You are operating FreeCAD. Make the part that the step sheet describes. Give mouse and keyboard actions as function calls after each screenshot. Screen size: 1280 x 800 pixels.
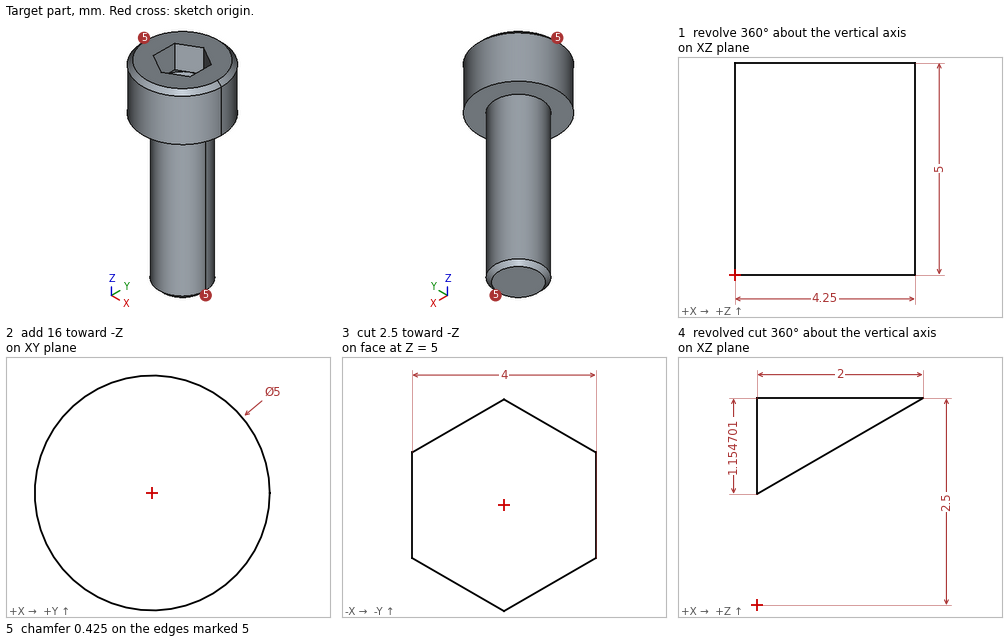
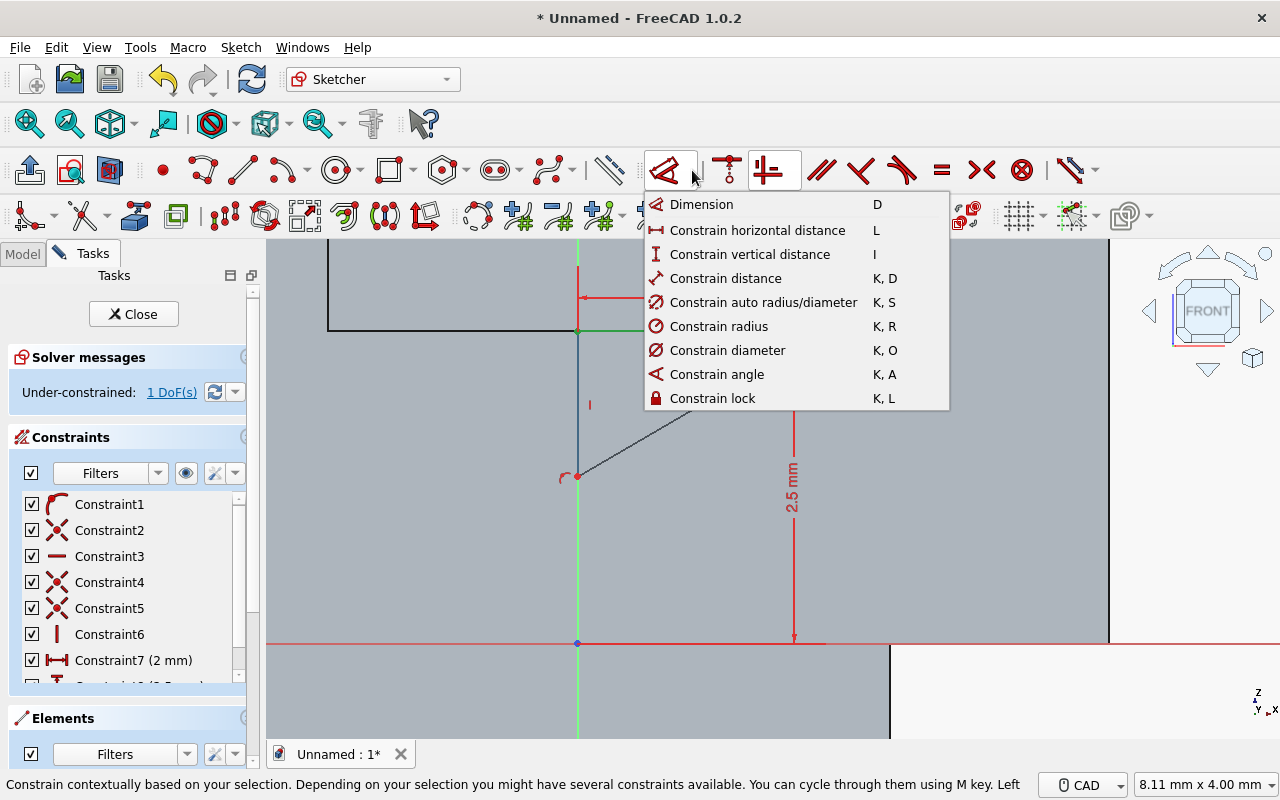
click(797, 254)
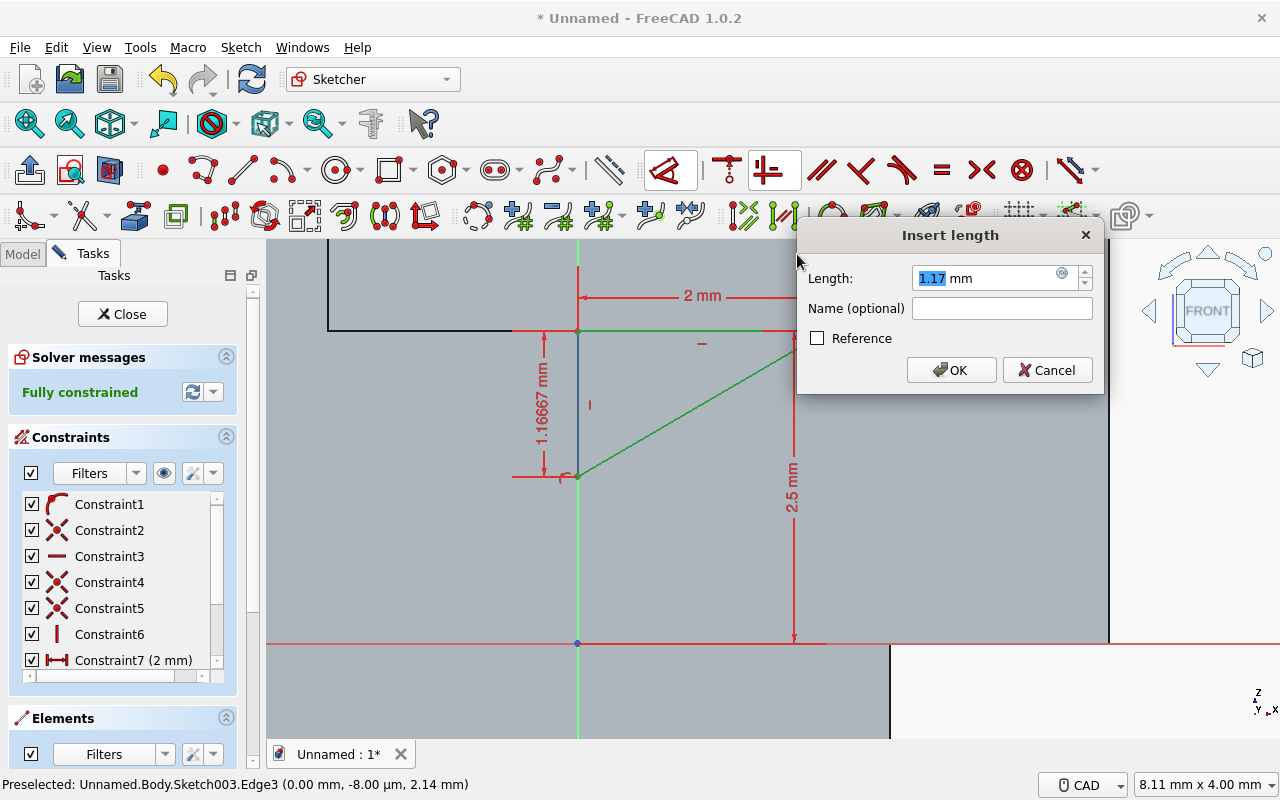
text(1.154701)
key(Return)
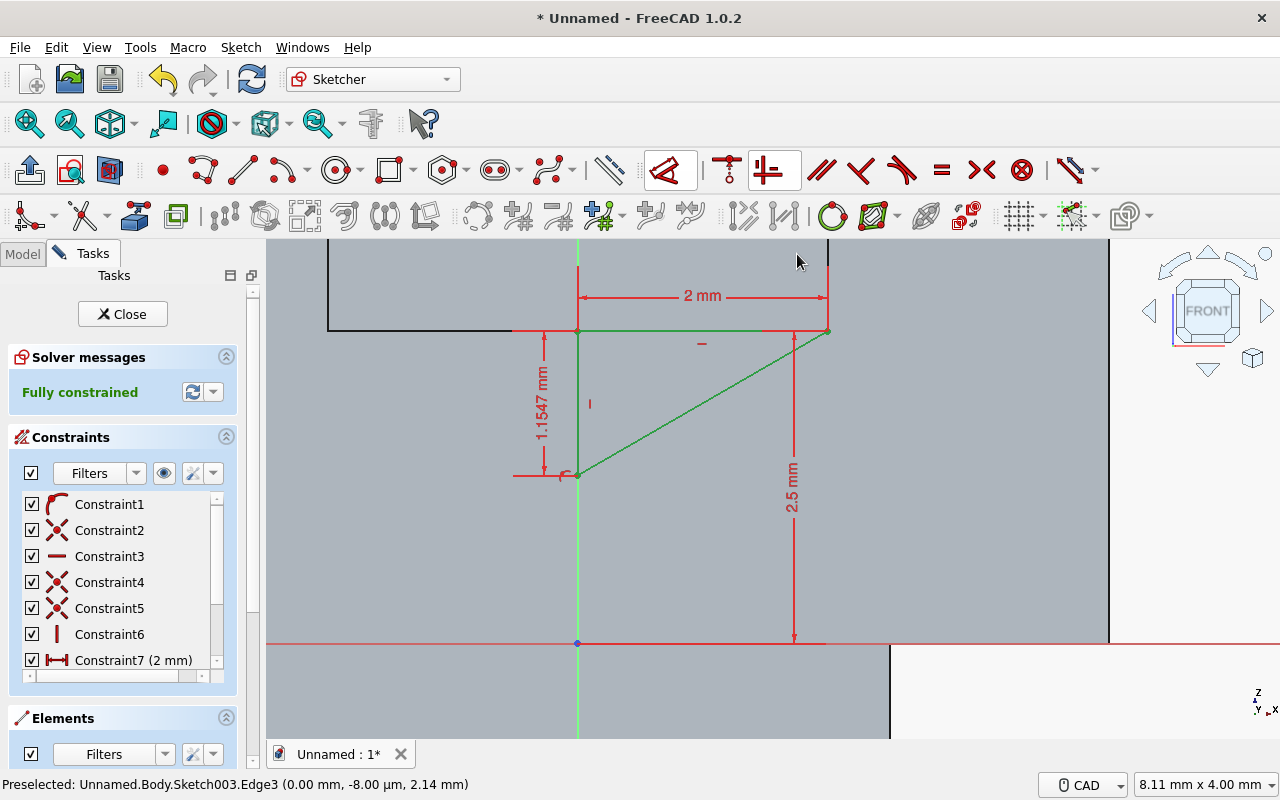
click(123, 314)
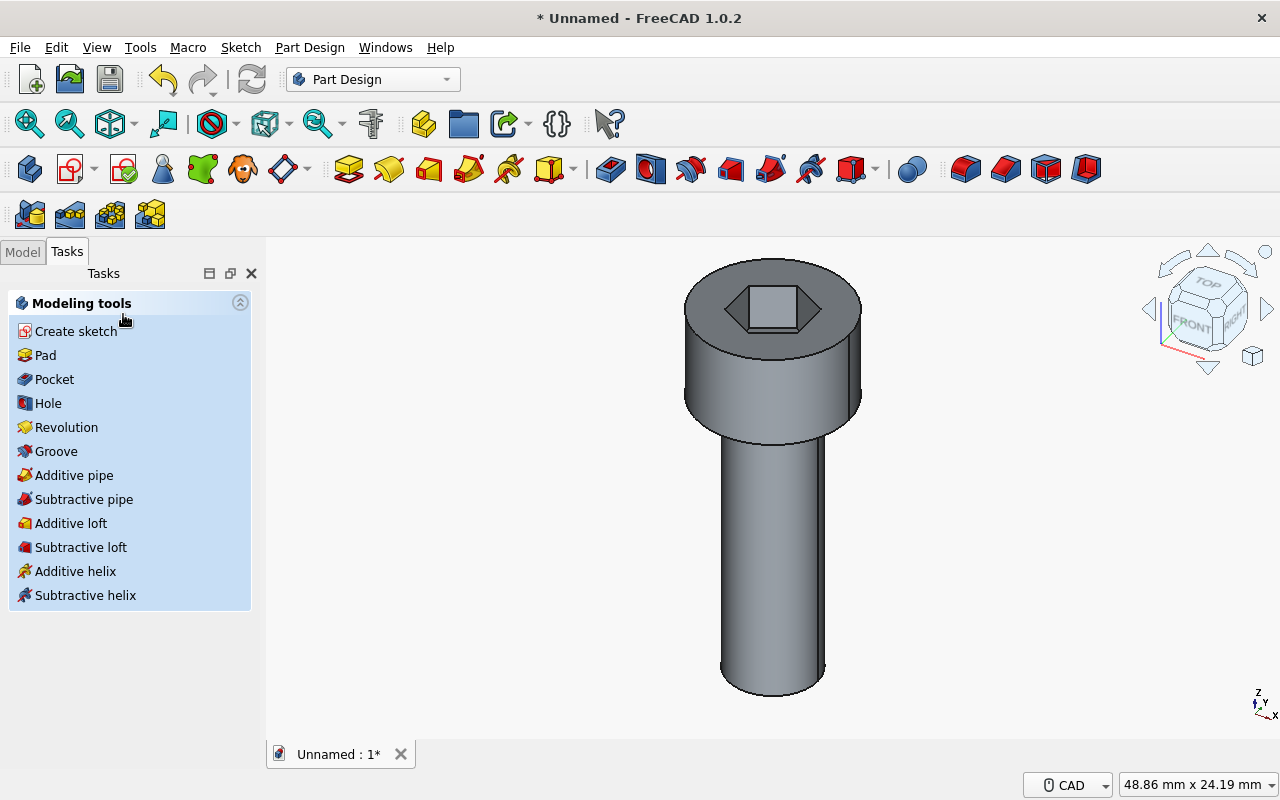
click(692, 170)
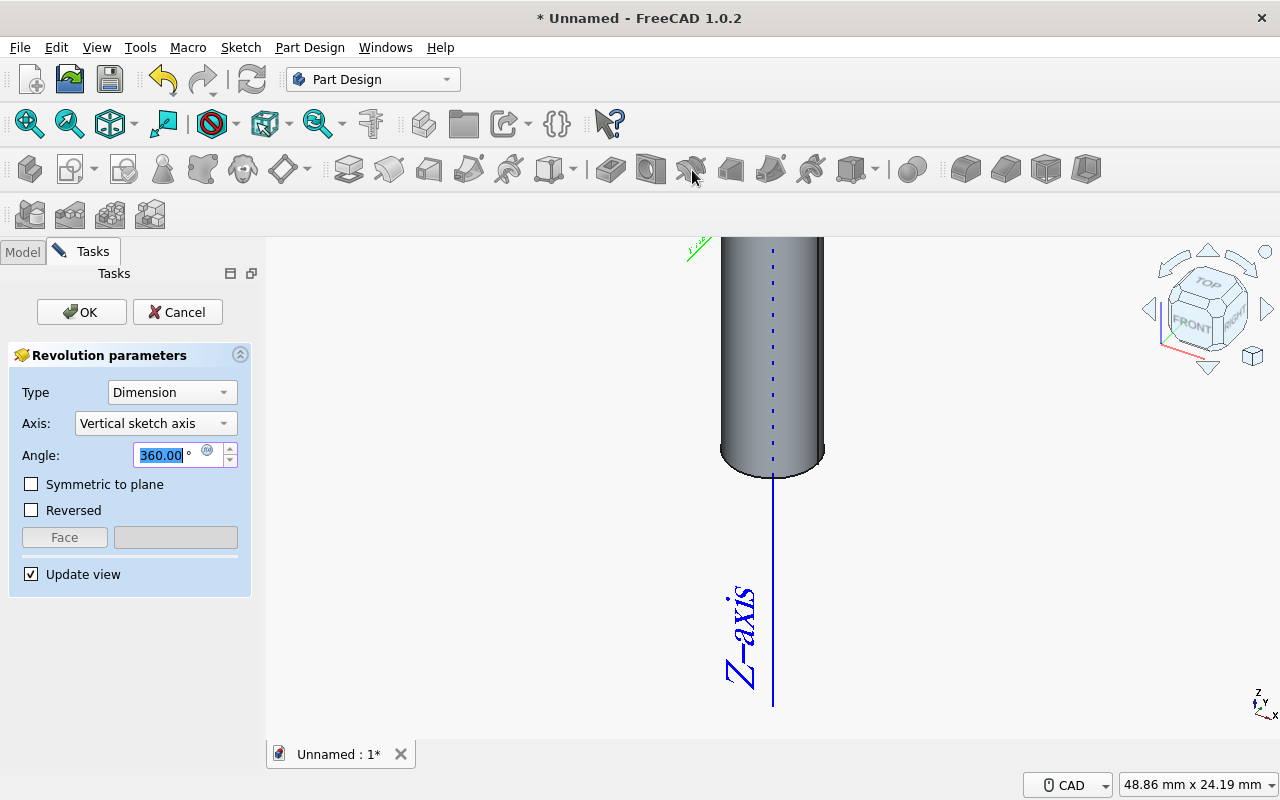
click(82, 312)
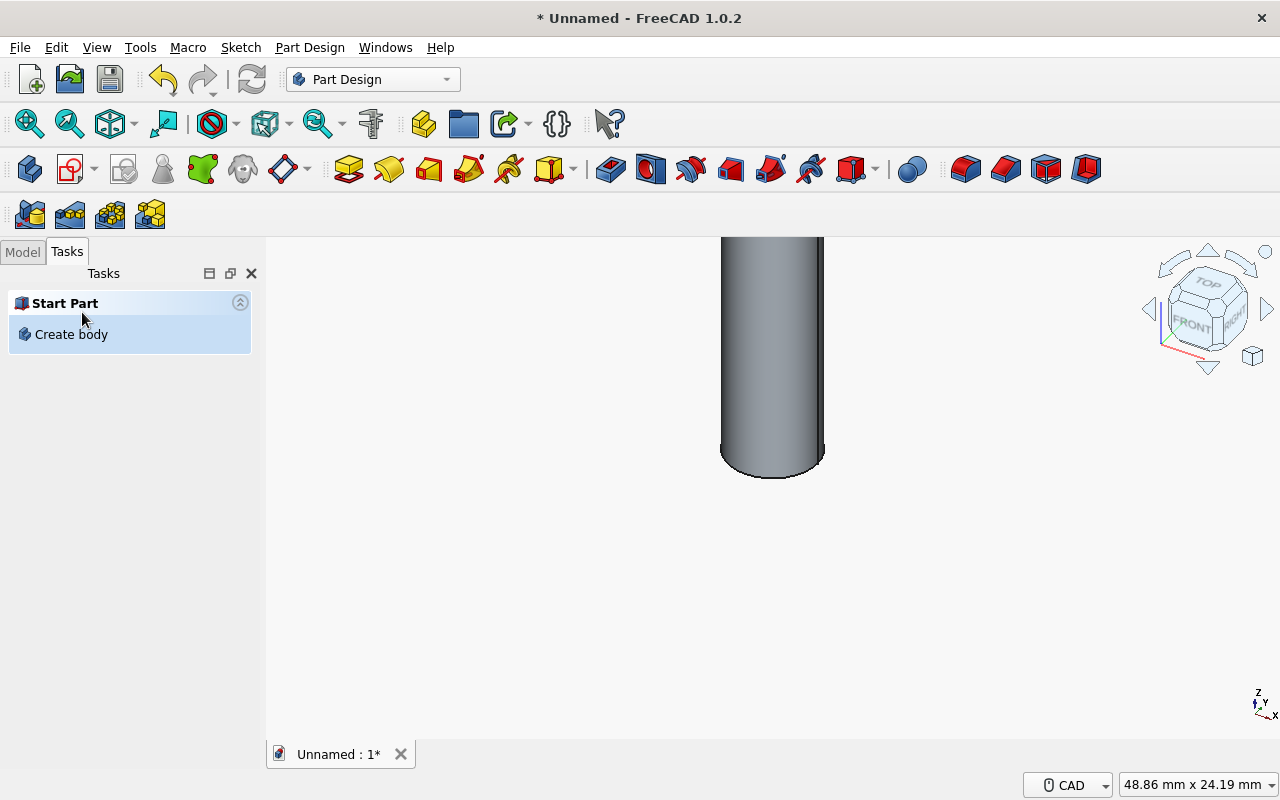
click(30, 124)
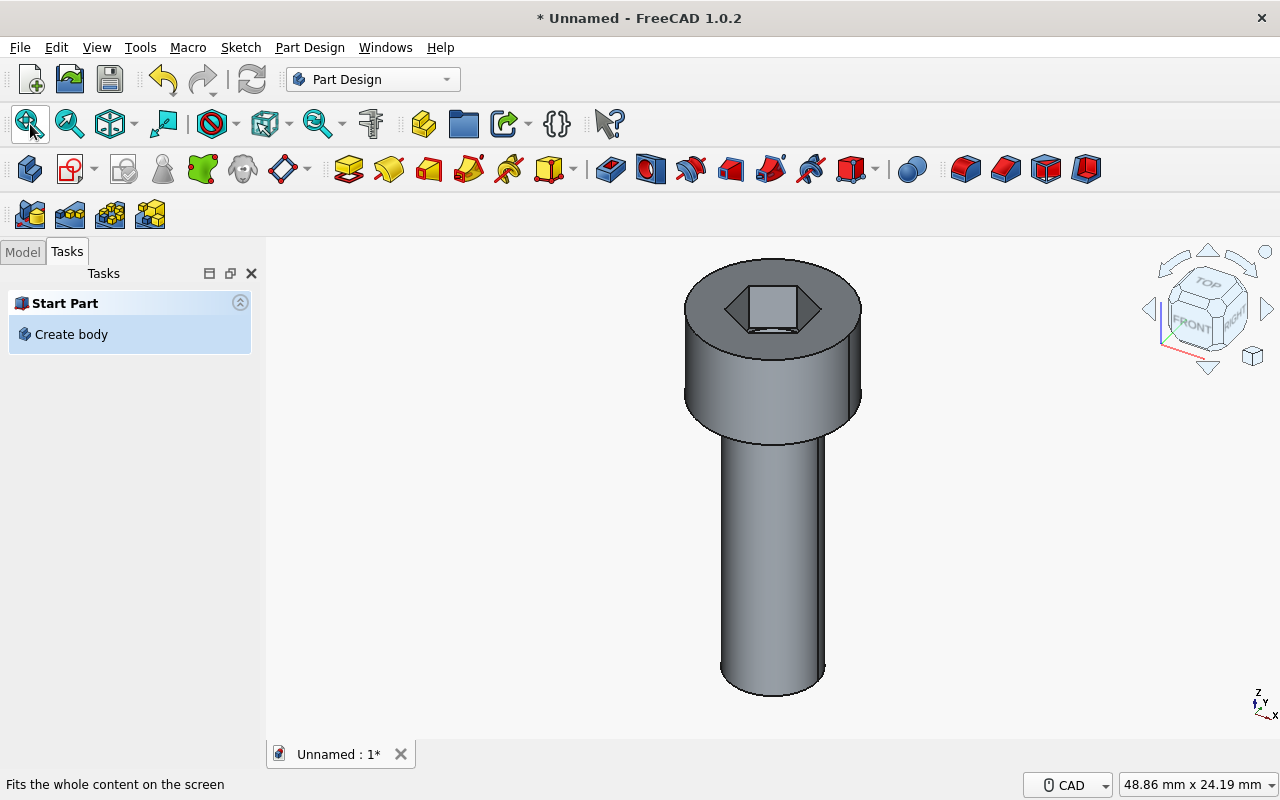
click(685, 314)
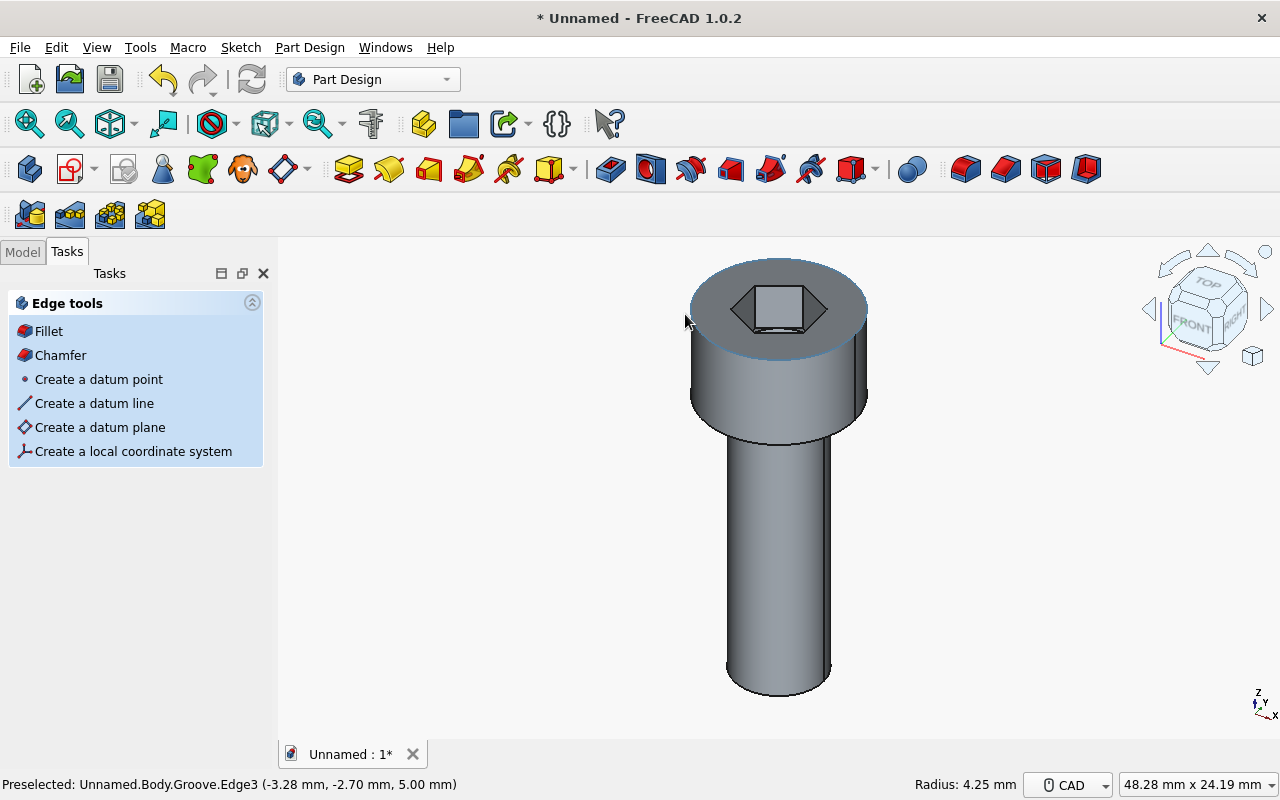
key(0)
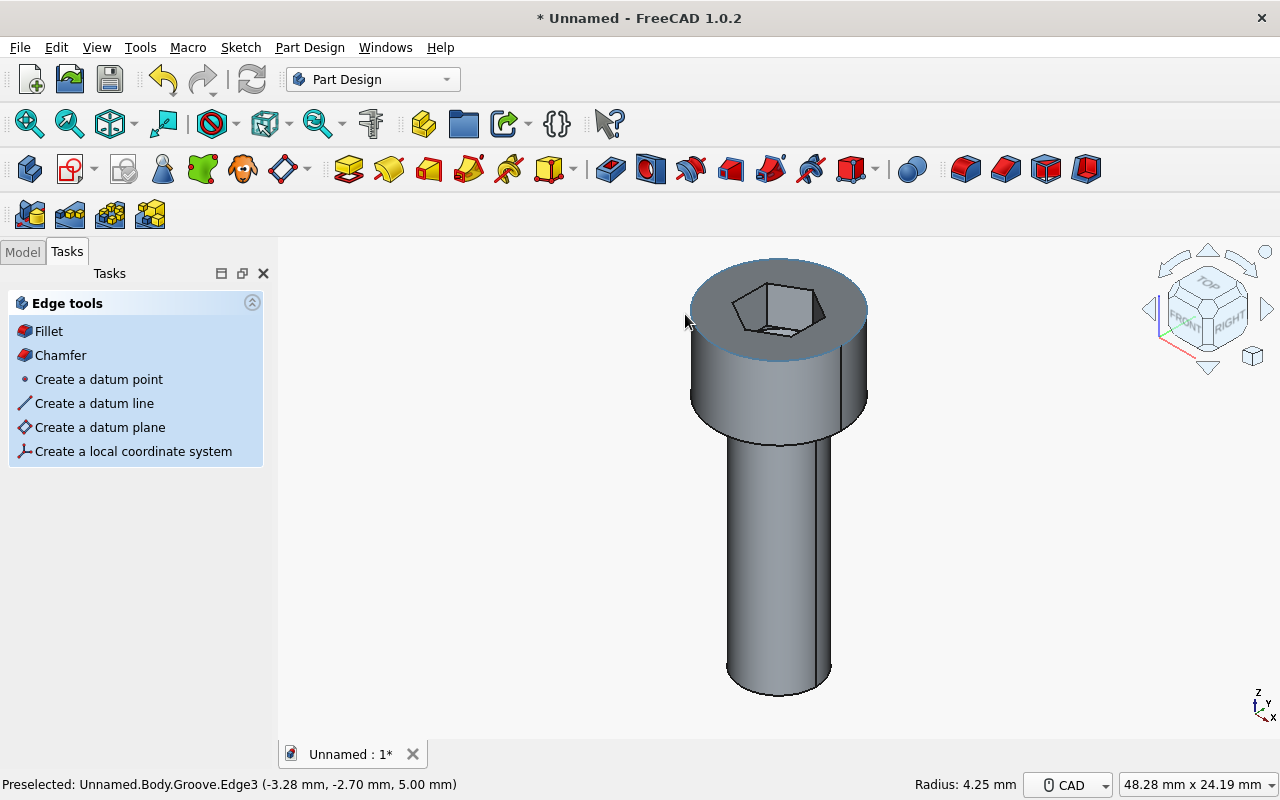
click(755, 692, ctrl)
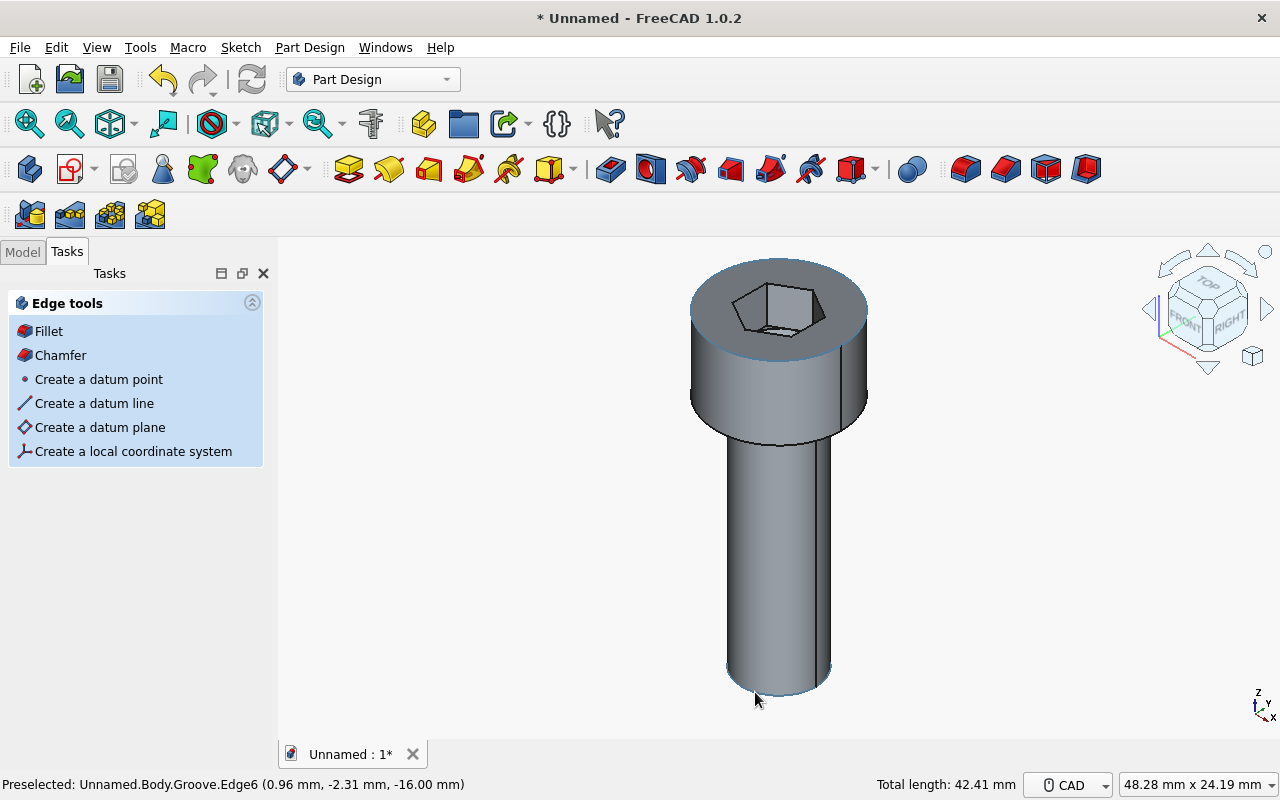
click(1006, 170)